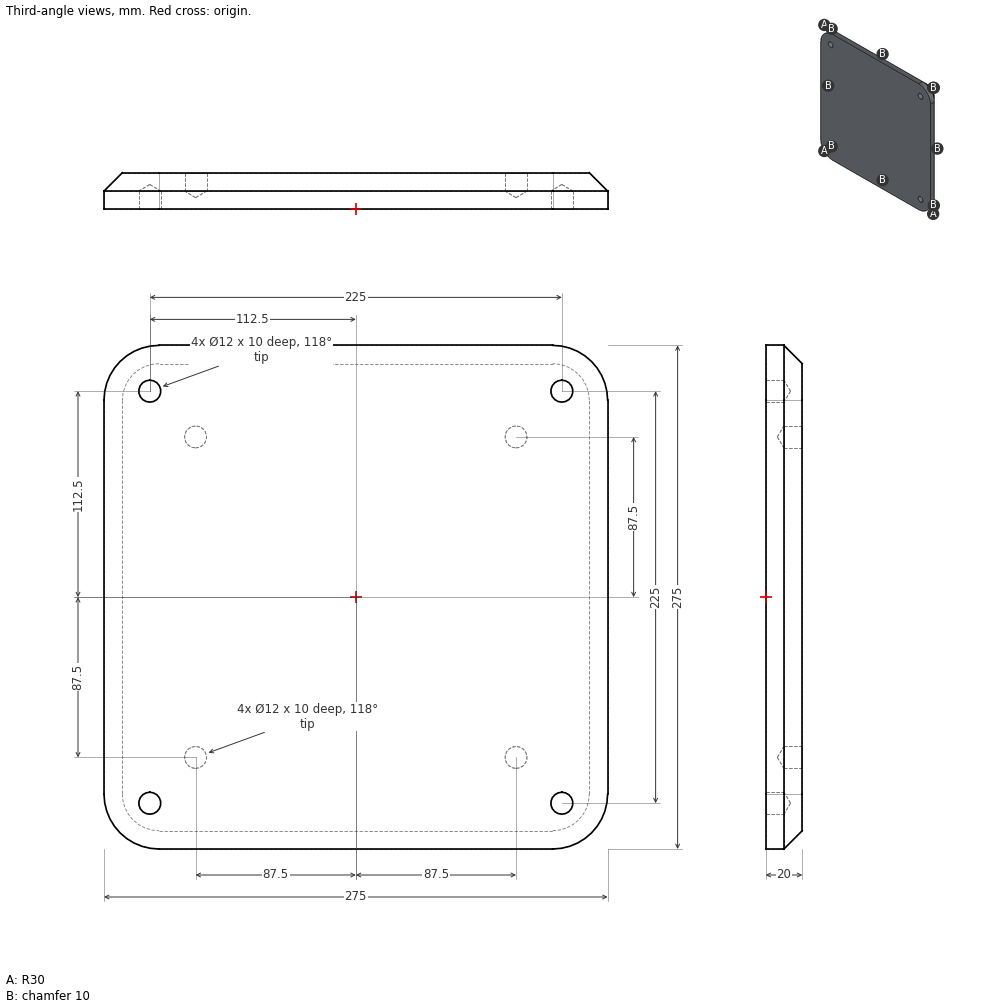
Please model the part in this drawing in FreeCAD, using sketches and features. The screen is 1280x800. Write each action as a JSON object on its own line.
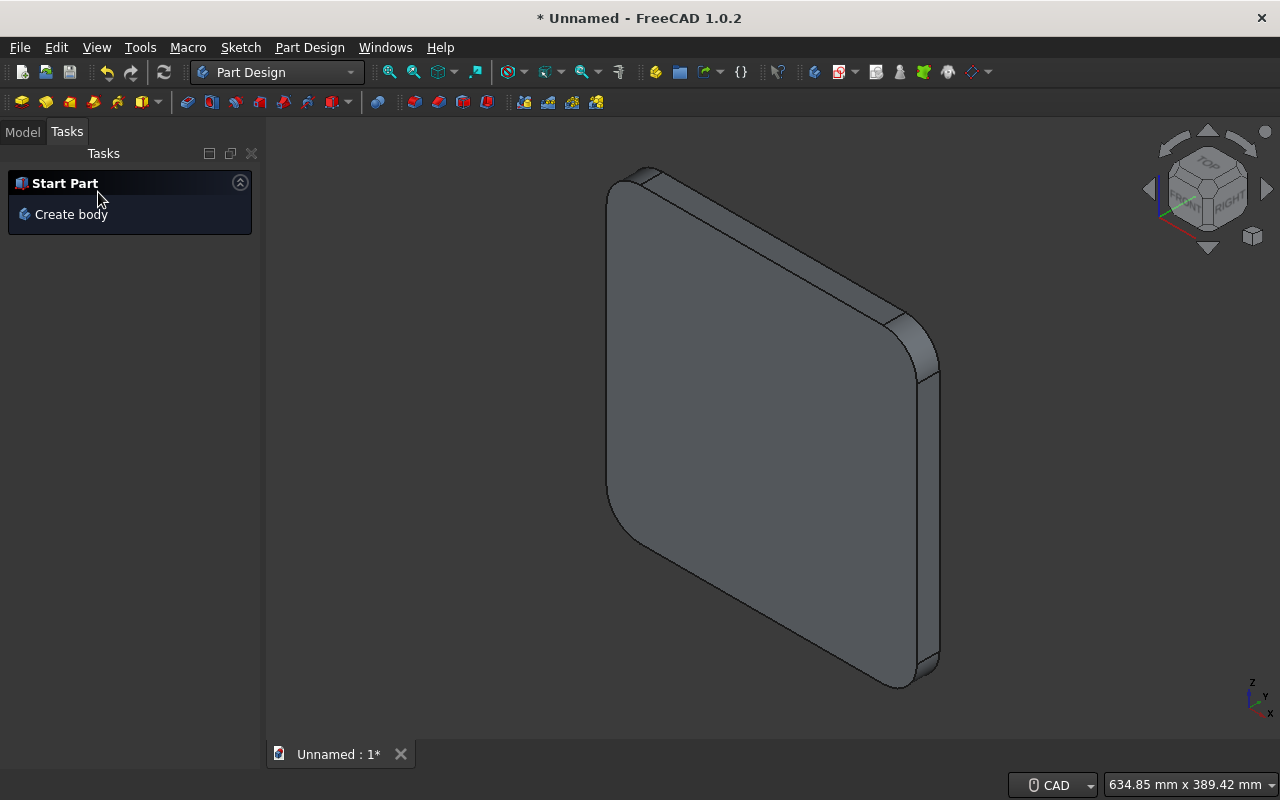
{"action": "key", "text": "2"}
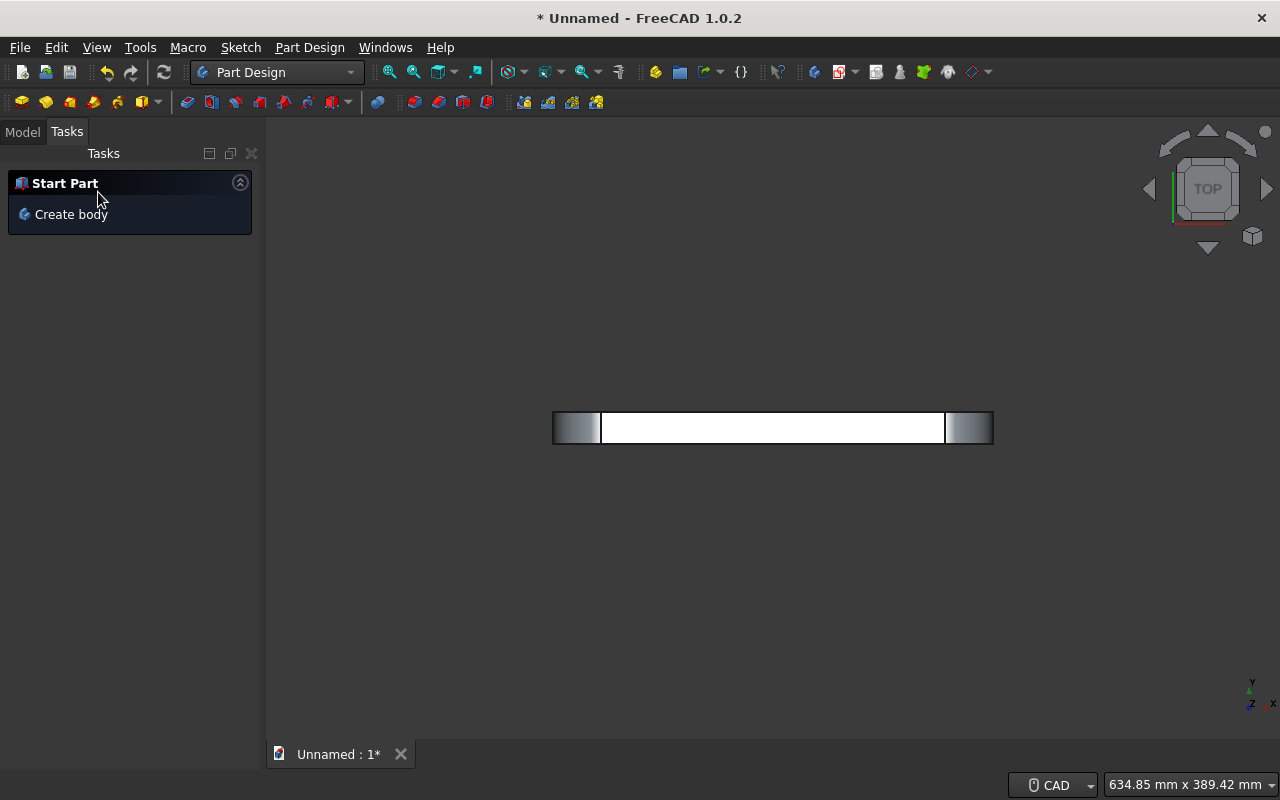
{"action": "left_click", "coordinate": [390, 72]}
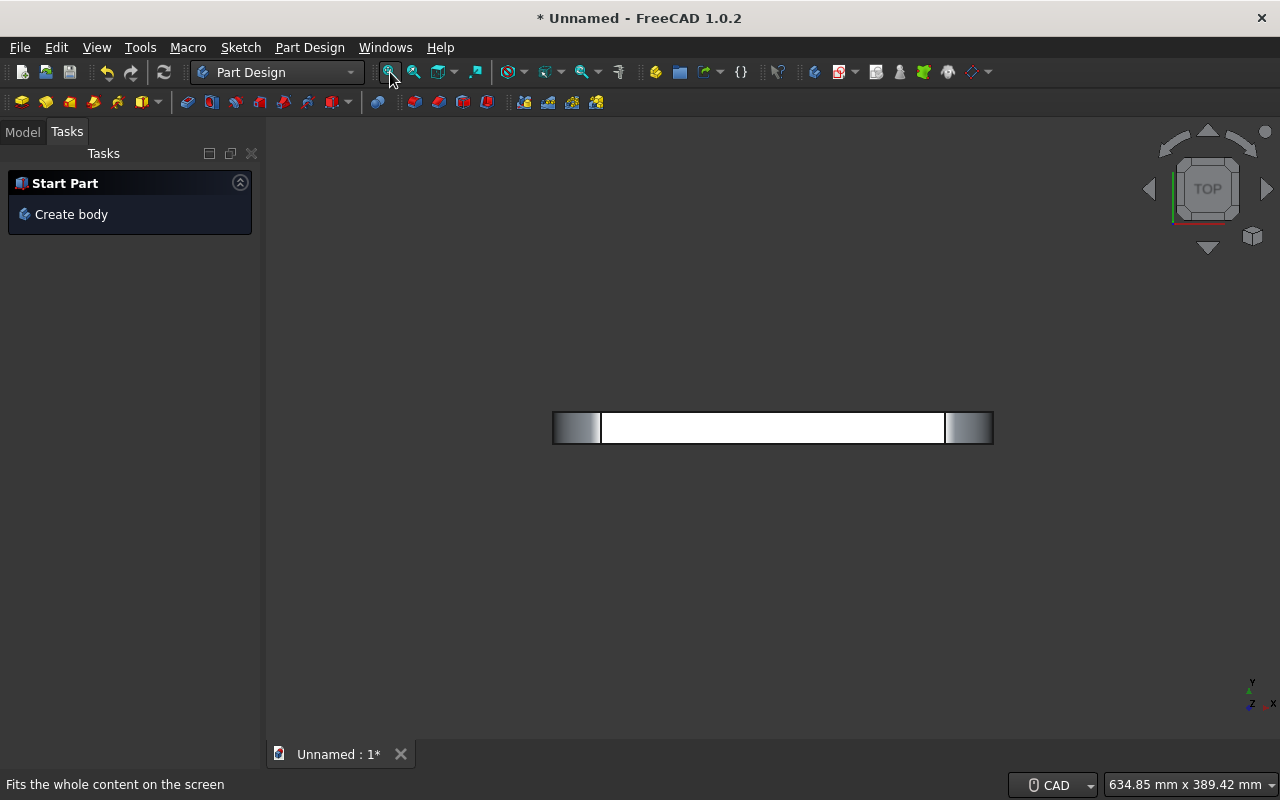
{"action": "key", "text": "1"}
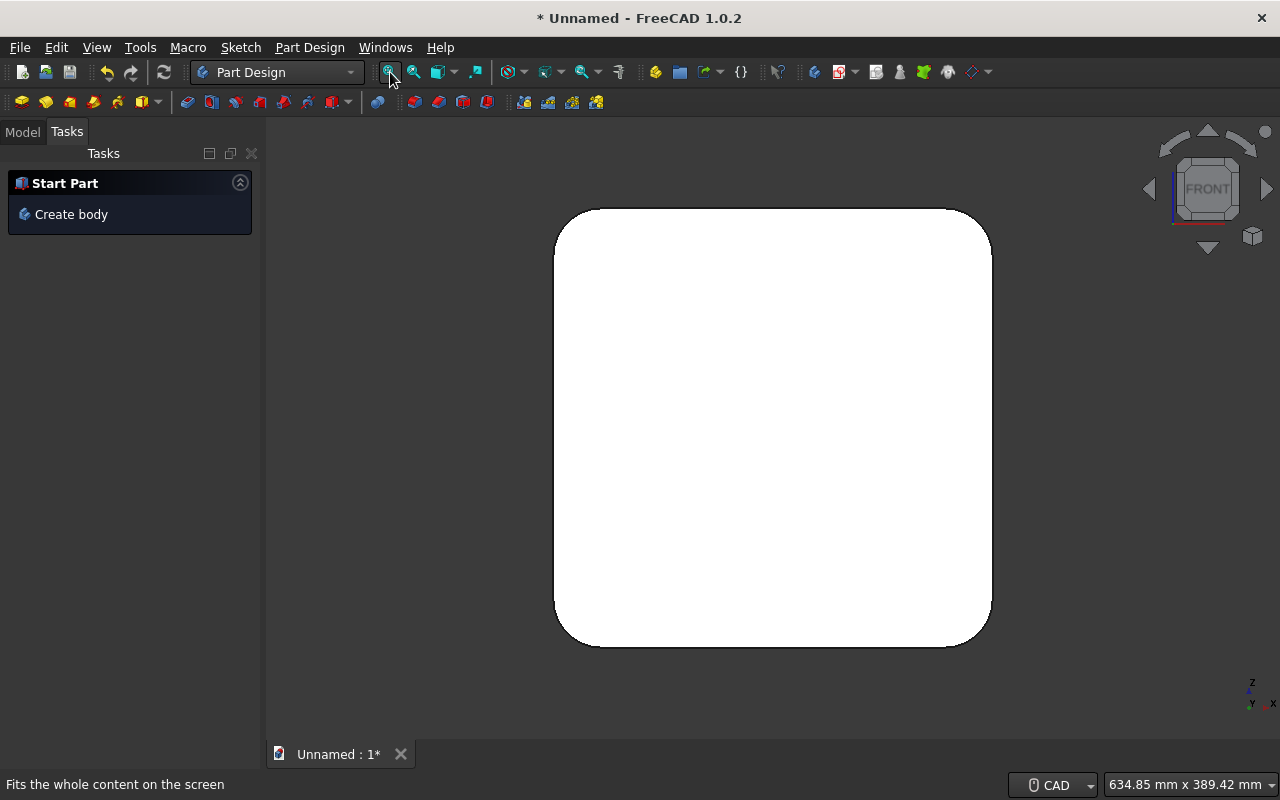
{"action": "key", "text": "3"}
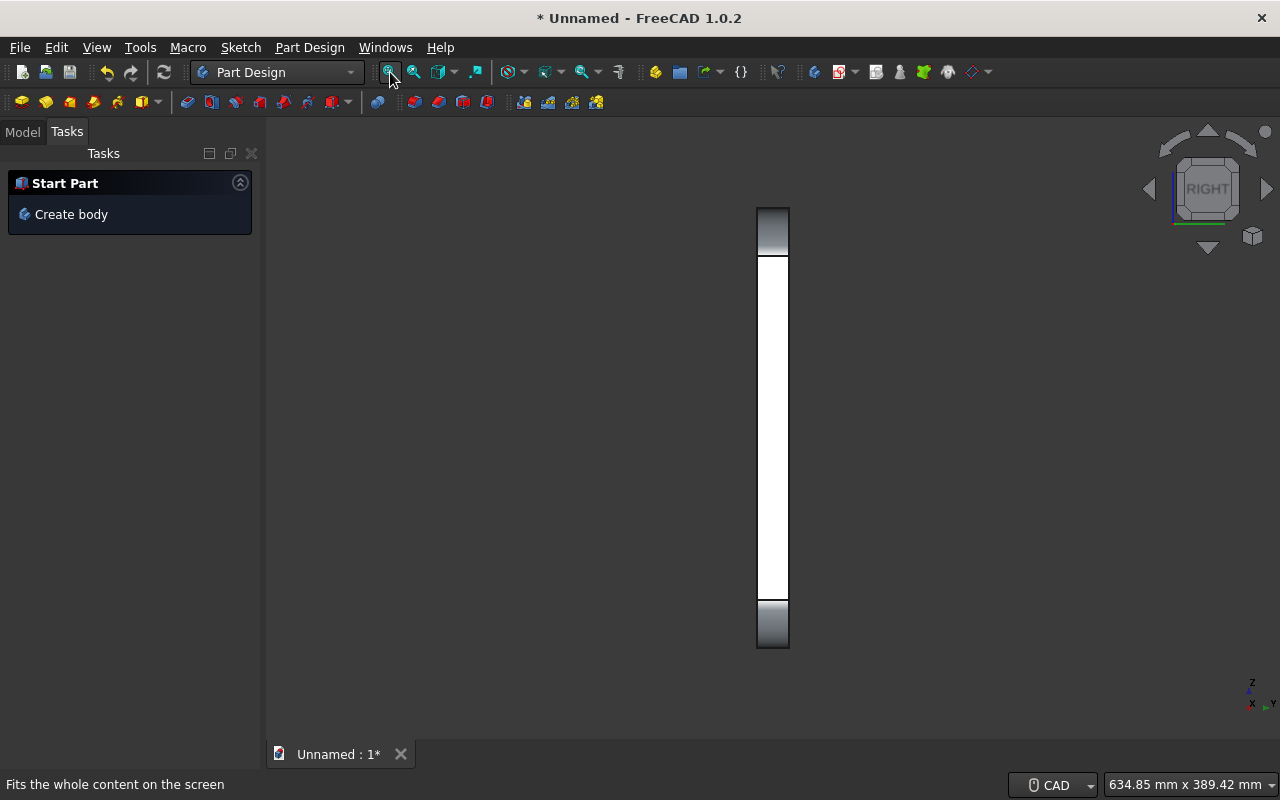
{"action": "key", "text": "5"}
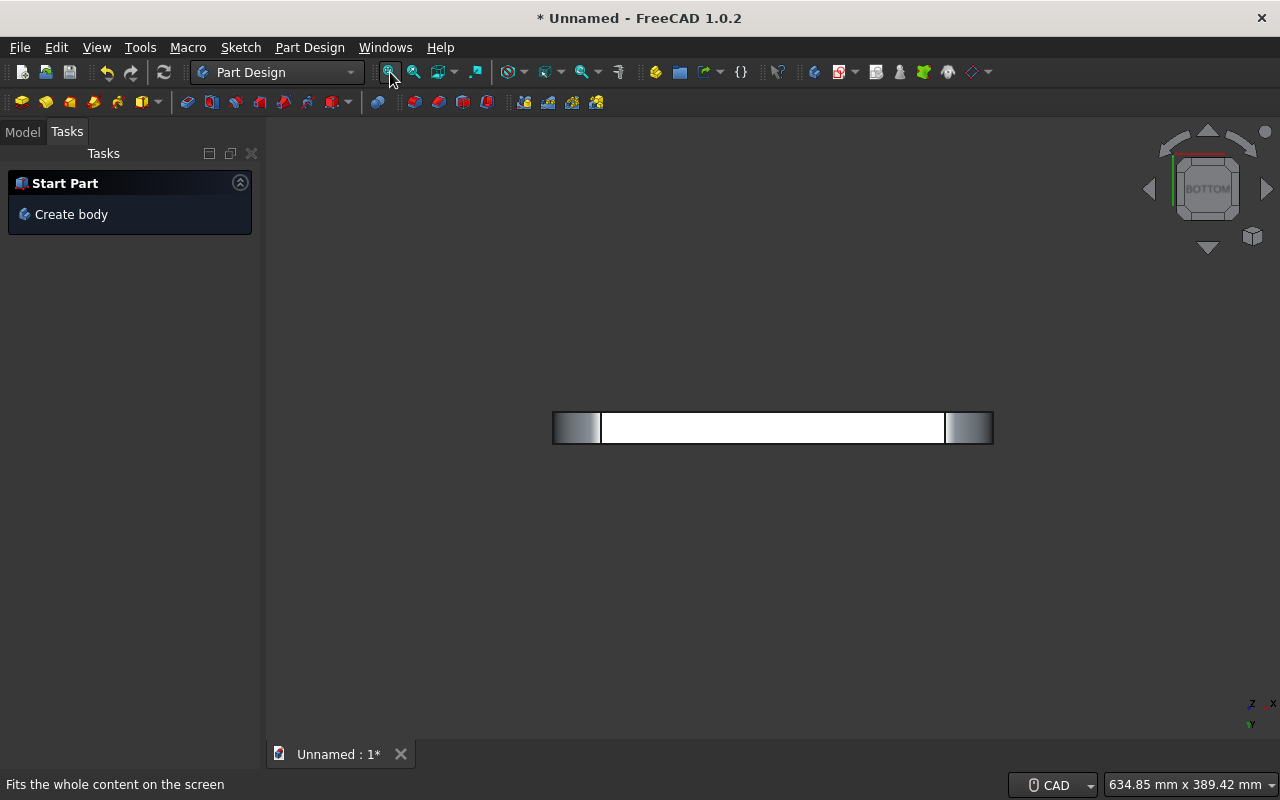
{"action": "key", "text": "v f"}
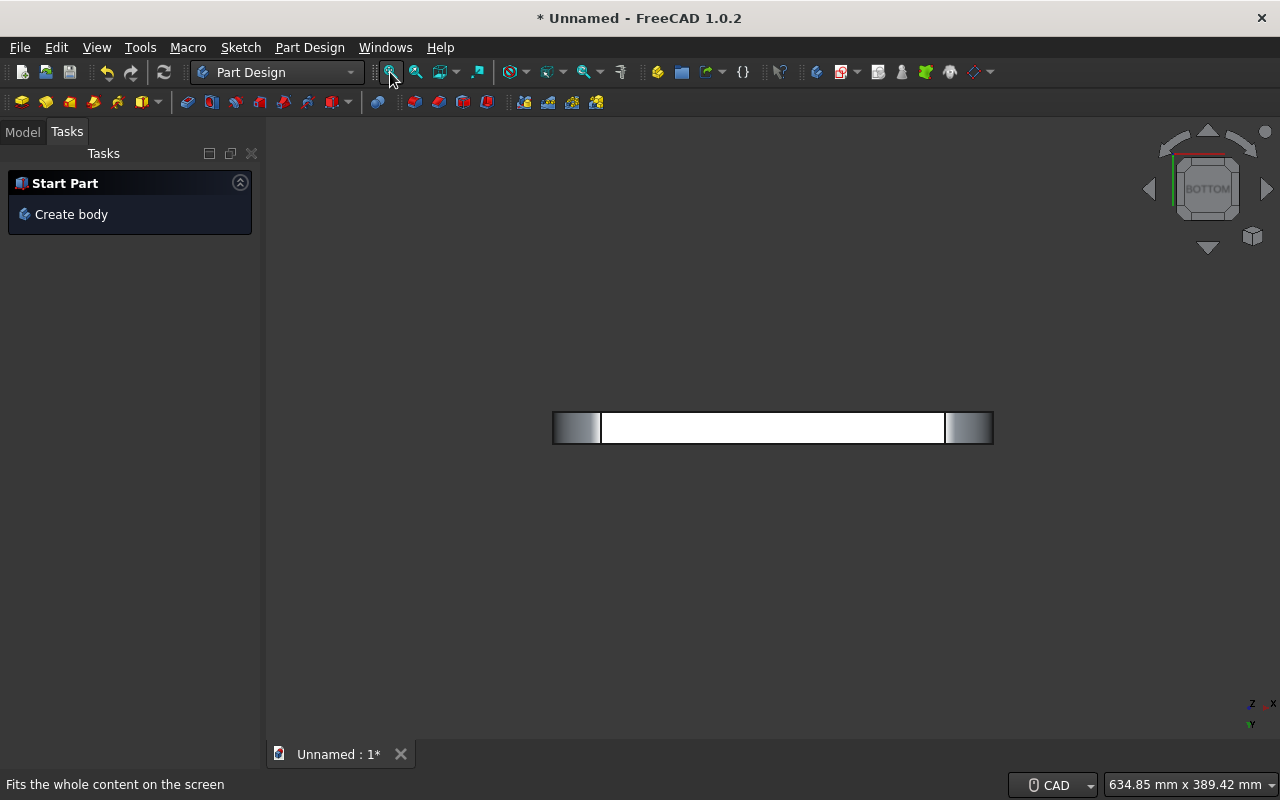
{"action": "key", "text": "4"}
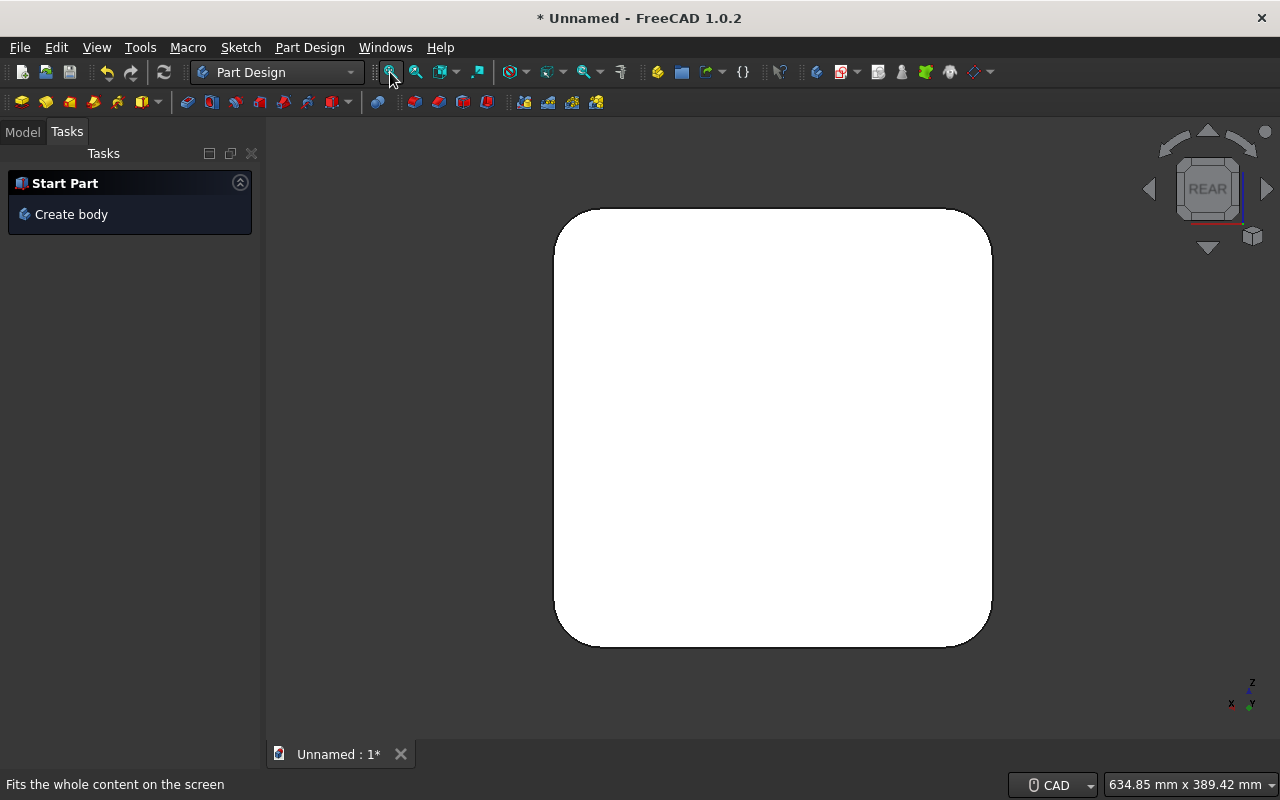
{"action": "left_click", "coordinate": [773, 427]}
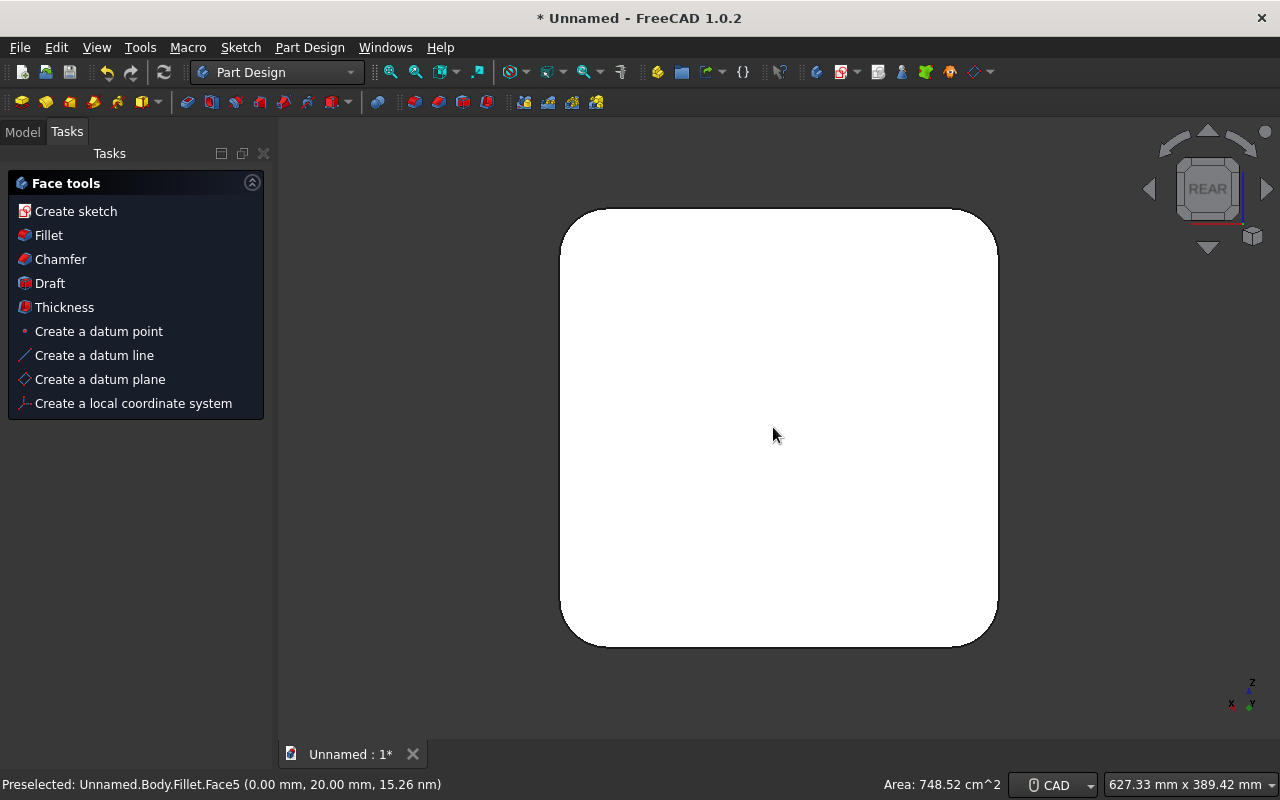
{"action": "left_click", "coordinate": [440, 102]}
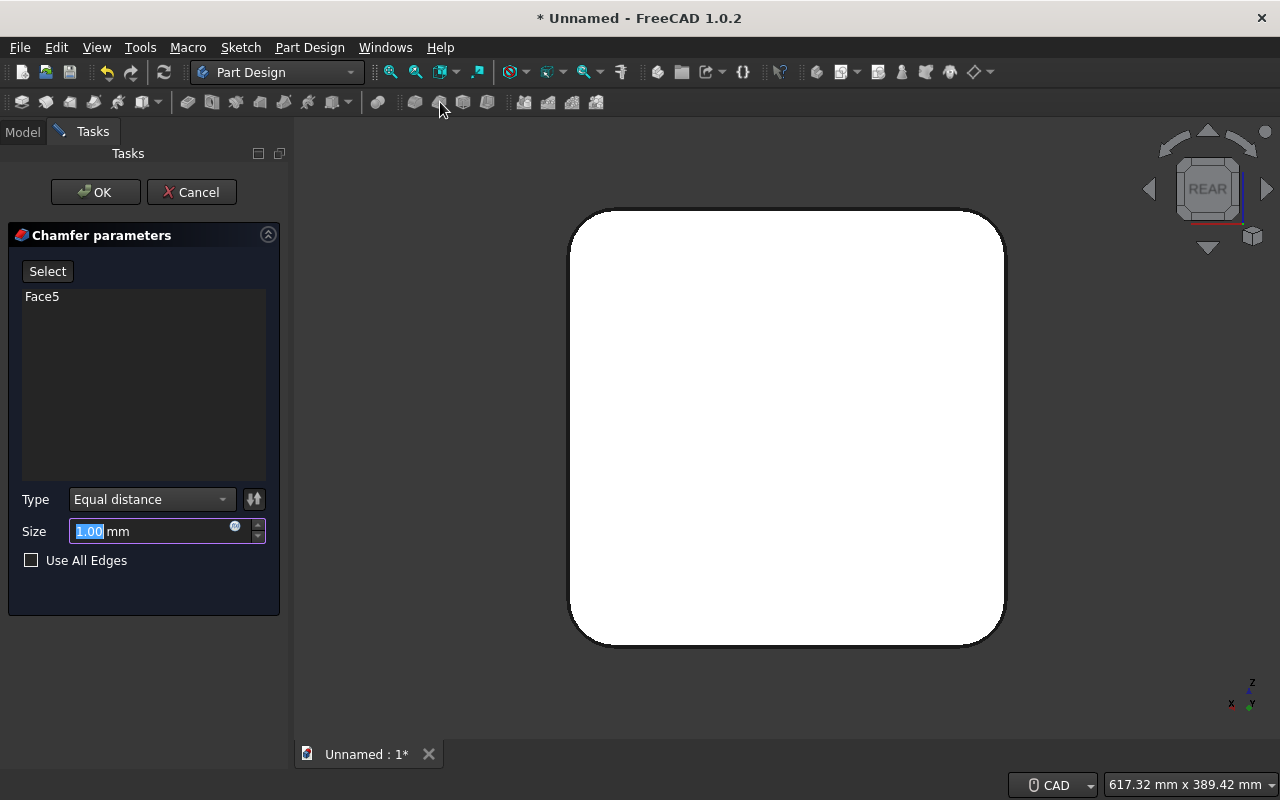
{"action": "type", "text": "10"}
{"action": "key", "text": "Tab"}